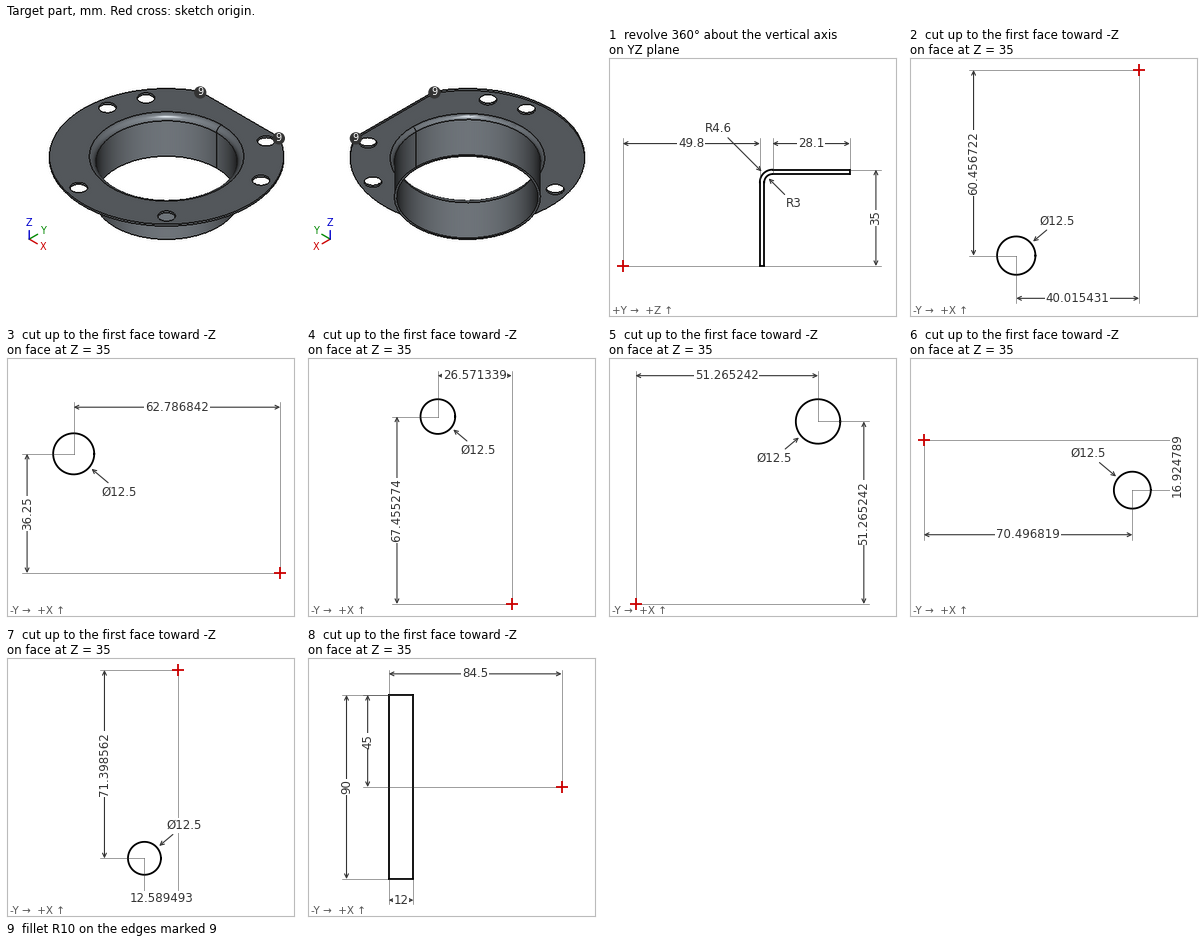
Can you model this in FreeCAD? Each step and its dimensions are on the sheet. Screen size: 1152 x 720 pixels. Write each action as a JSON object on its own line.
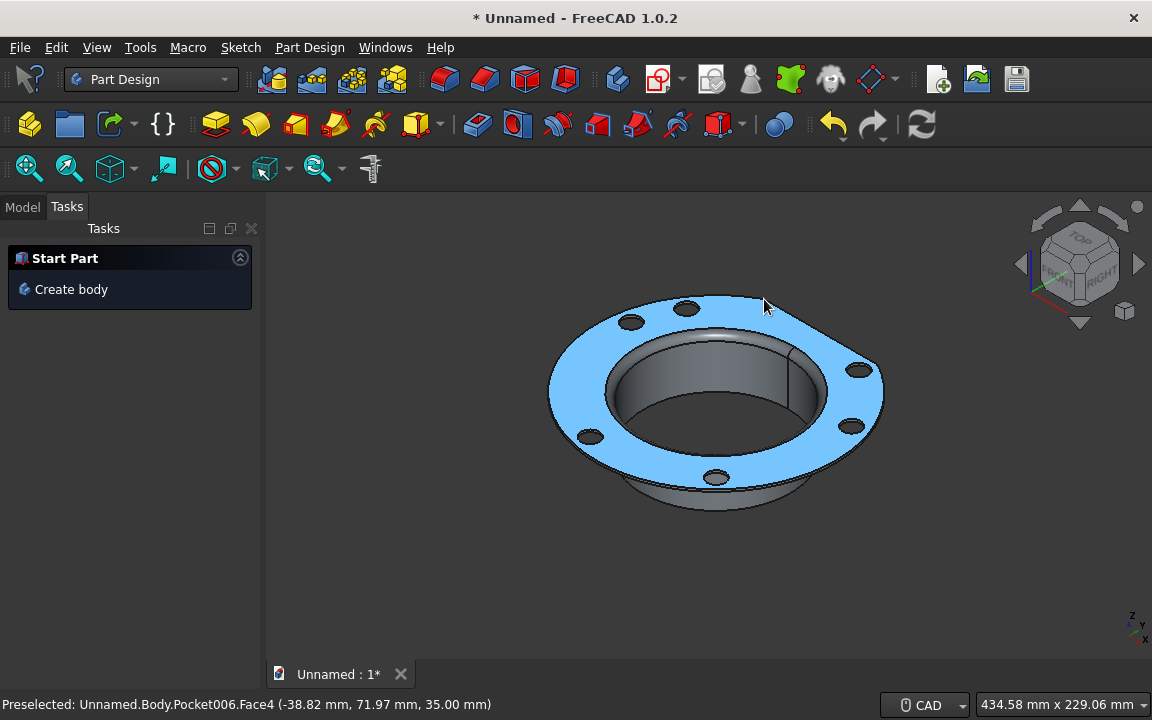
{"action": "key", "text": "2"}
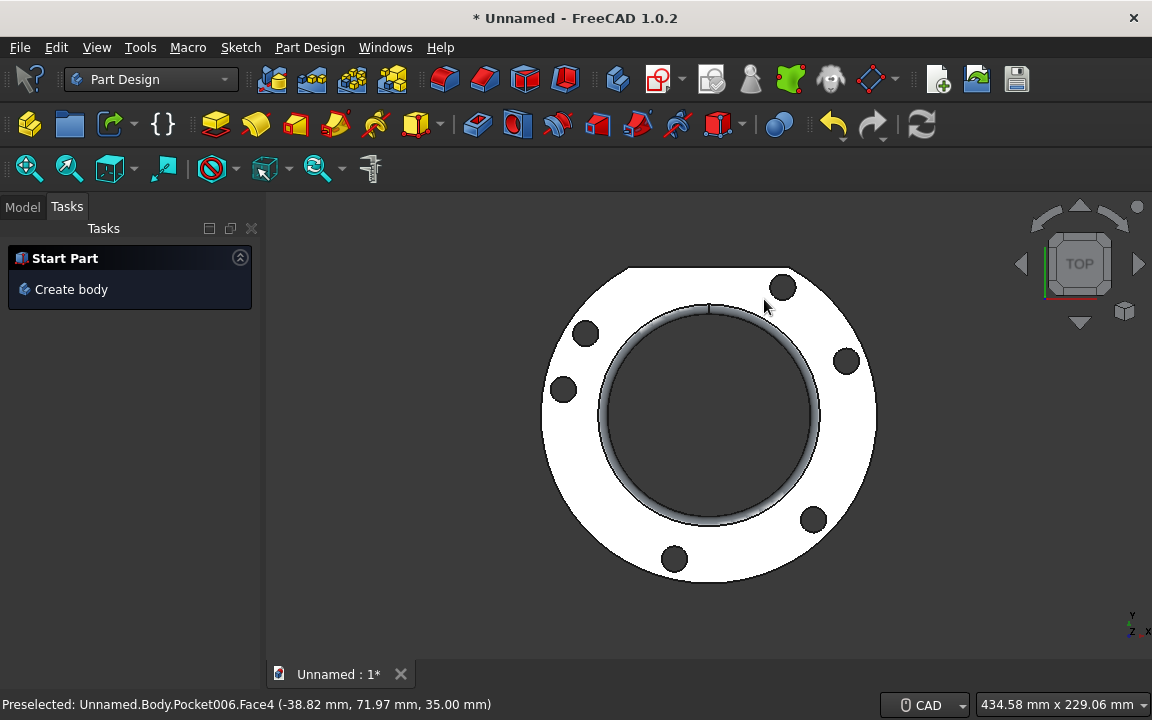
{"action": "scroll", "coordinate": [629, 266], "scroll_direction": "up", "scroll_amount": 13}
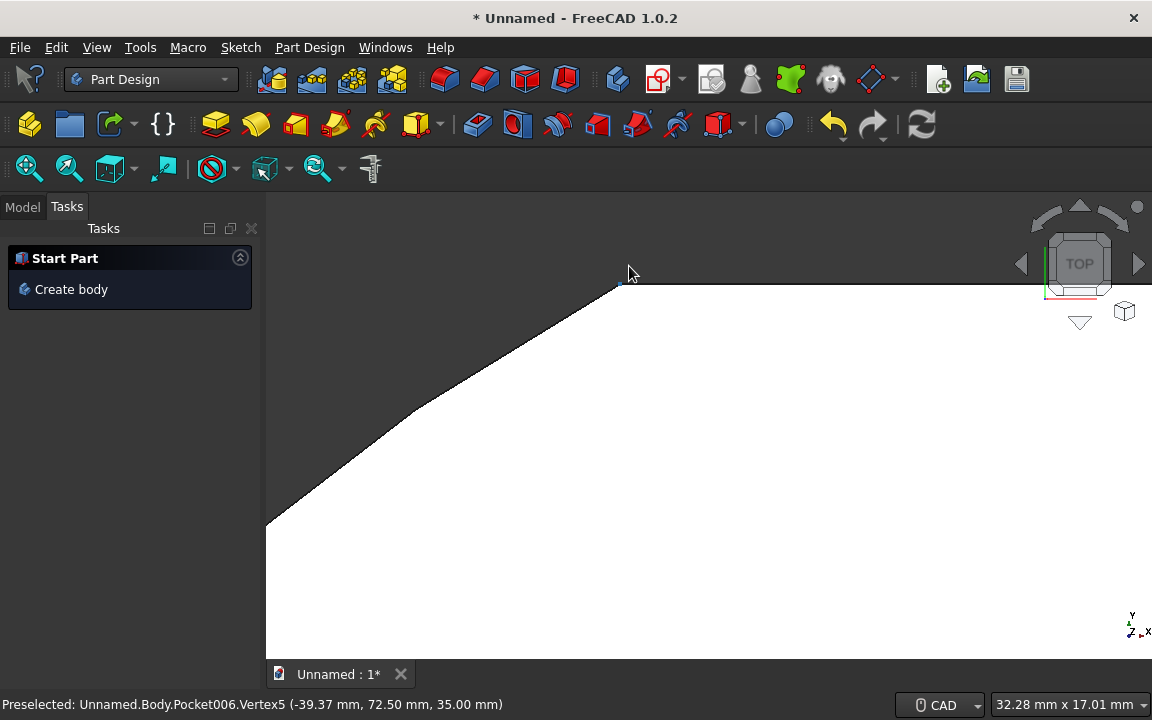
{"action": "key", "text": "v f"}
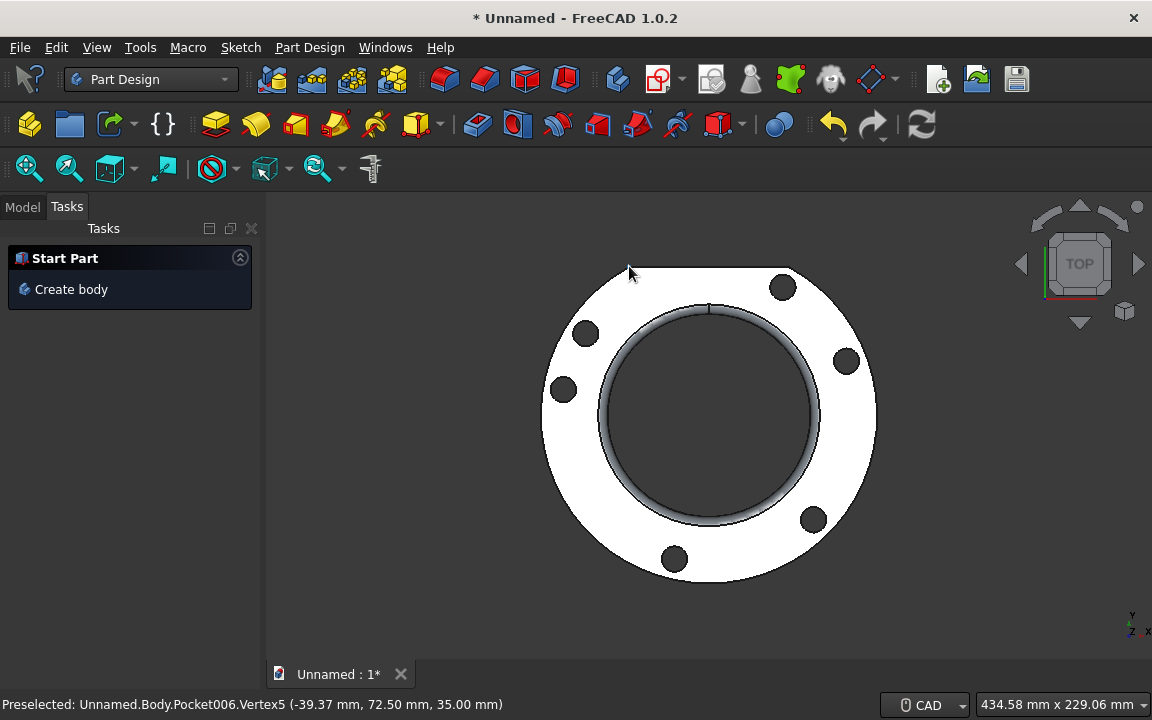
{"action": "key", "text": "1"}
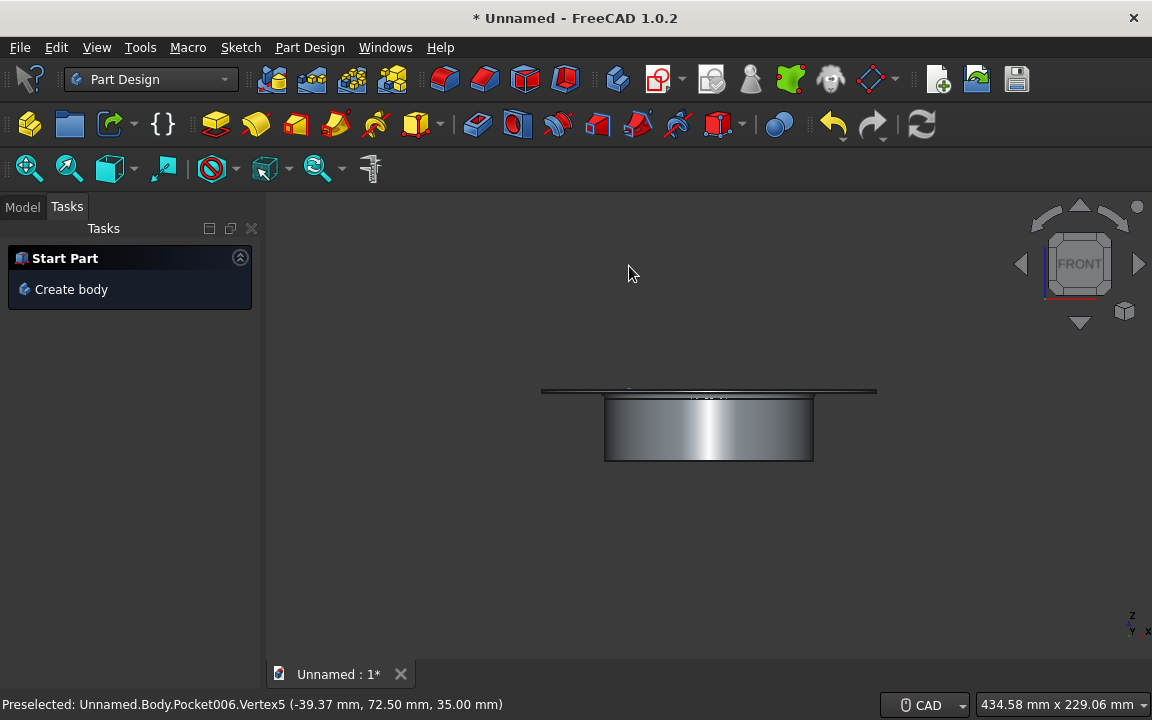
{"action": "left_click", "coordinate": [30, 170]}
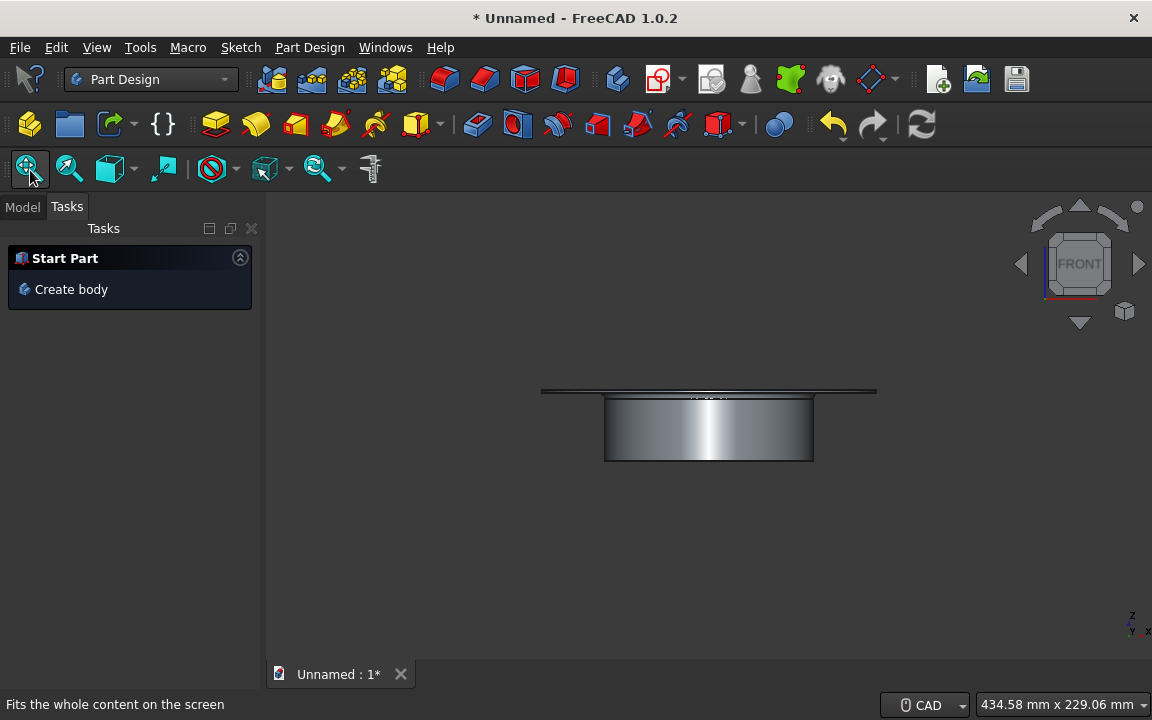
{"action": "scroll", "coordinate": [629, 390], "scroll_direction": "up", "scroll_amount": 13}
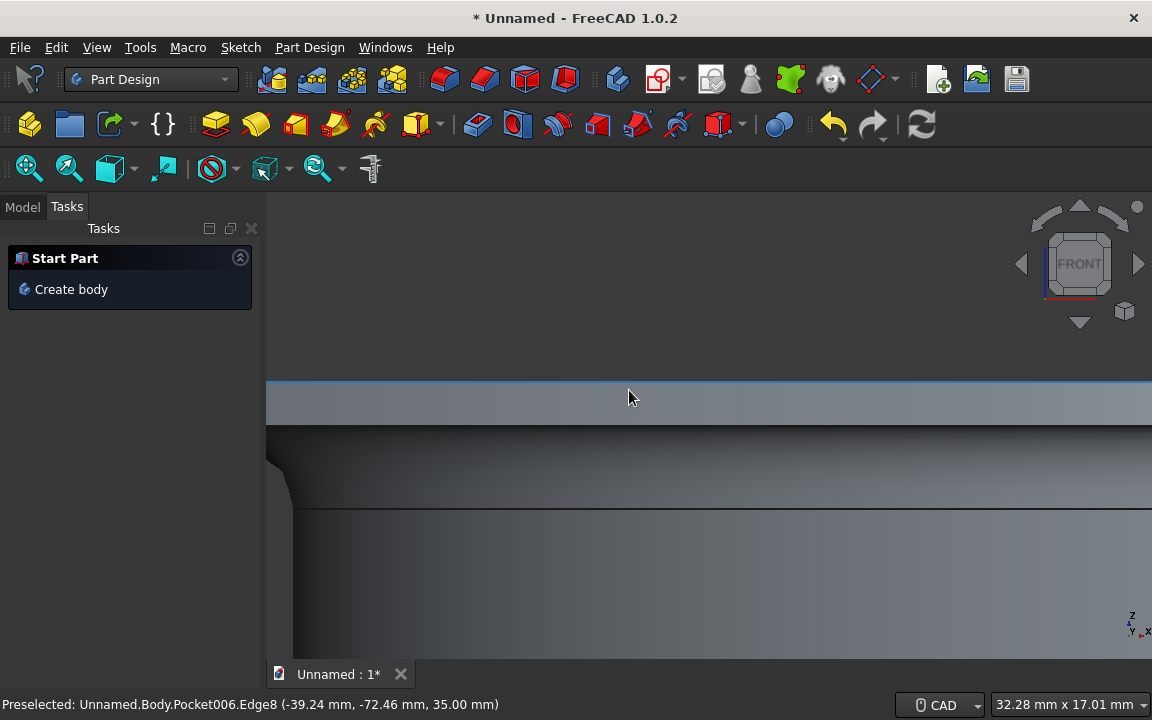
{"action": "key", "text": "v f"}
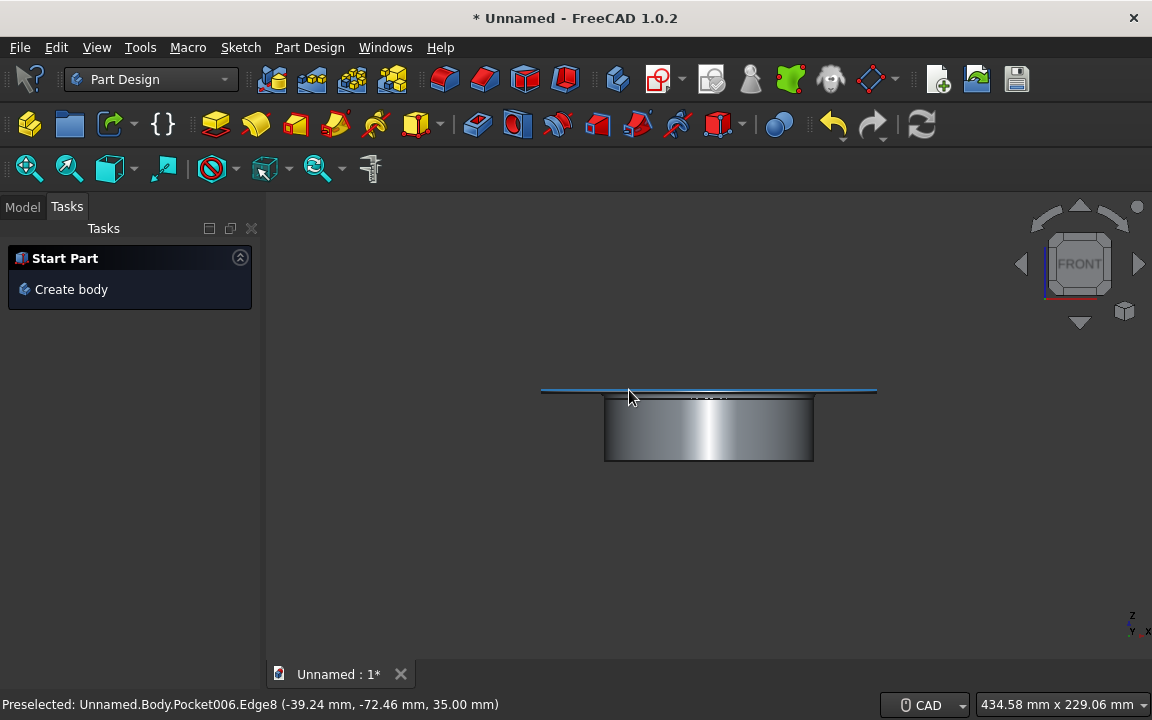
{"action": "key", "text": "3"}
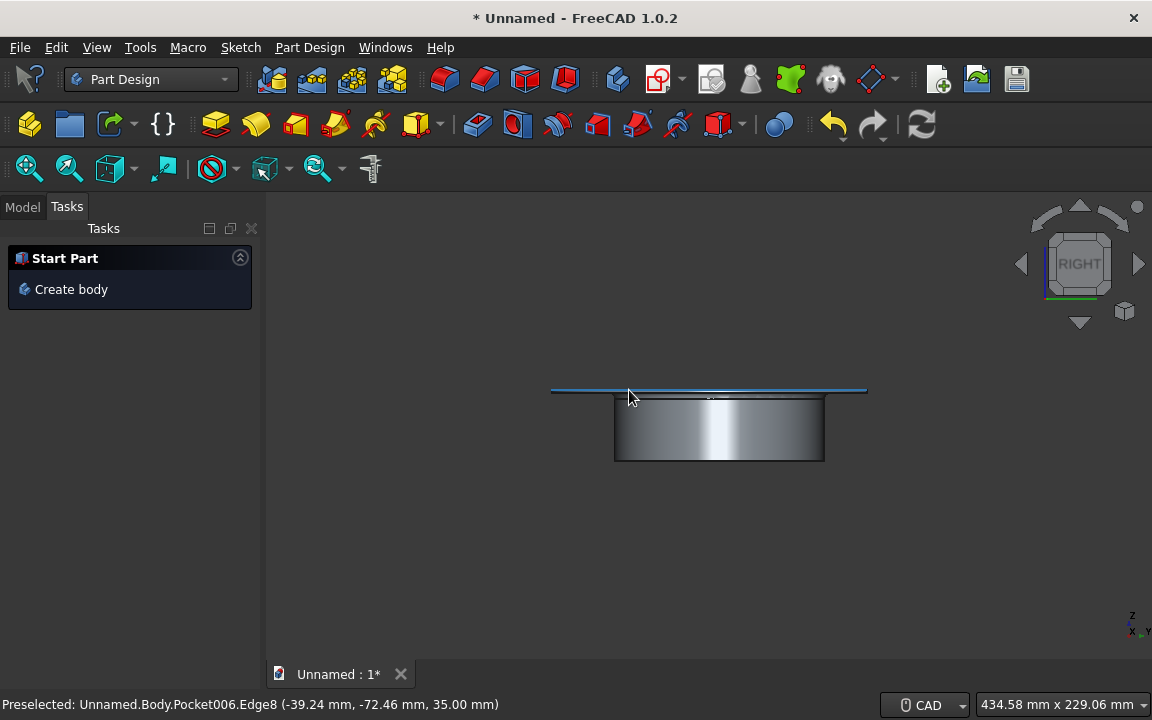
{"action": "key", "text": "v f"}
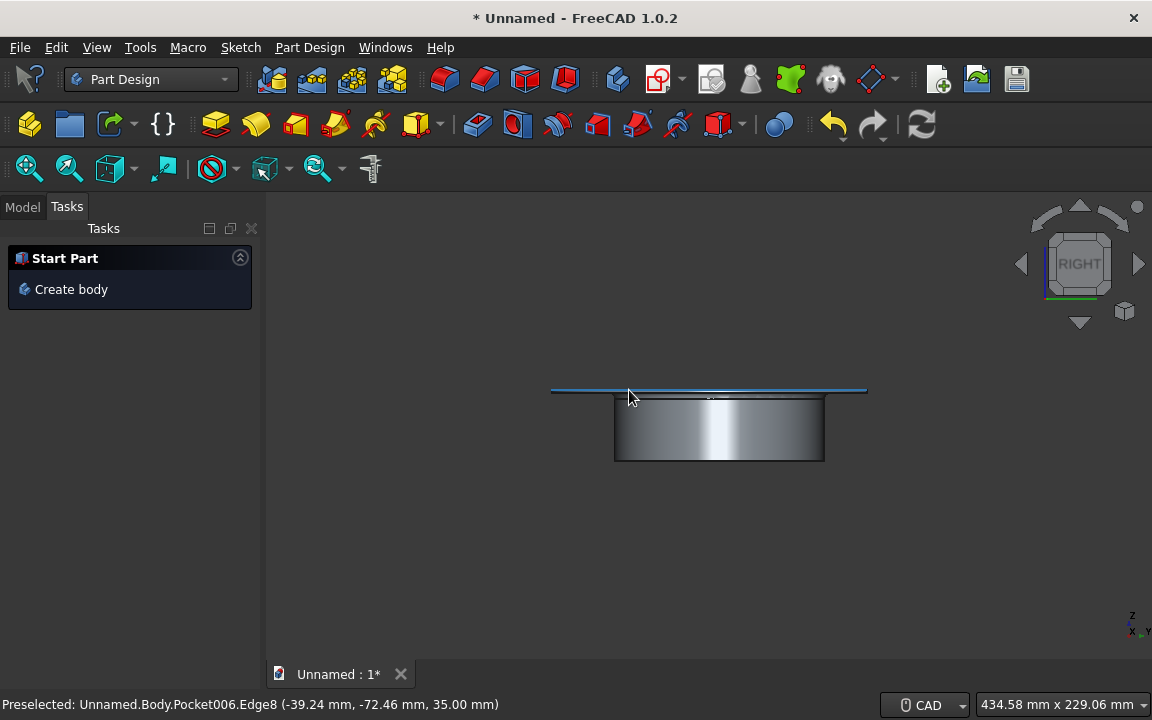
{"action": "scroll", "coordinate": [867, 390], "scroll_direction": "up", "scroll_amount": 13}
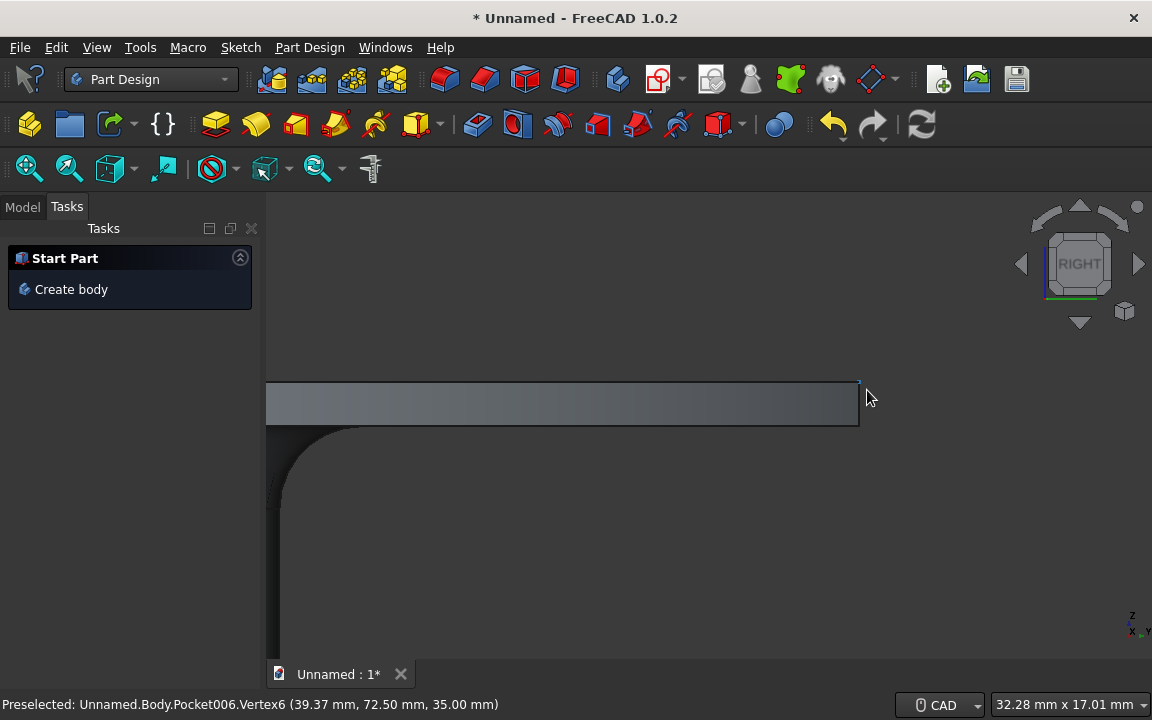
{"action": "key", "text": "v f"}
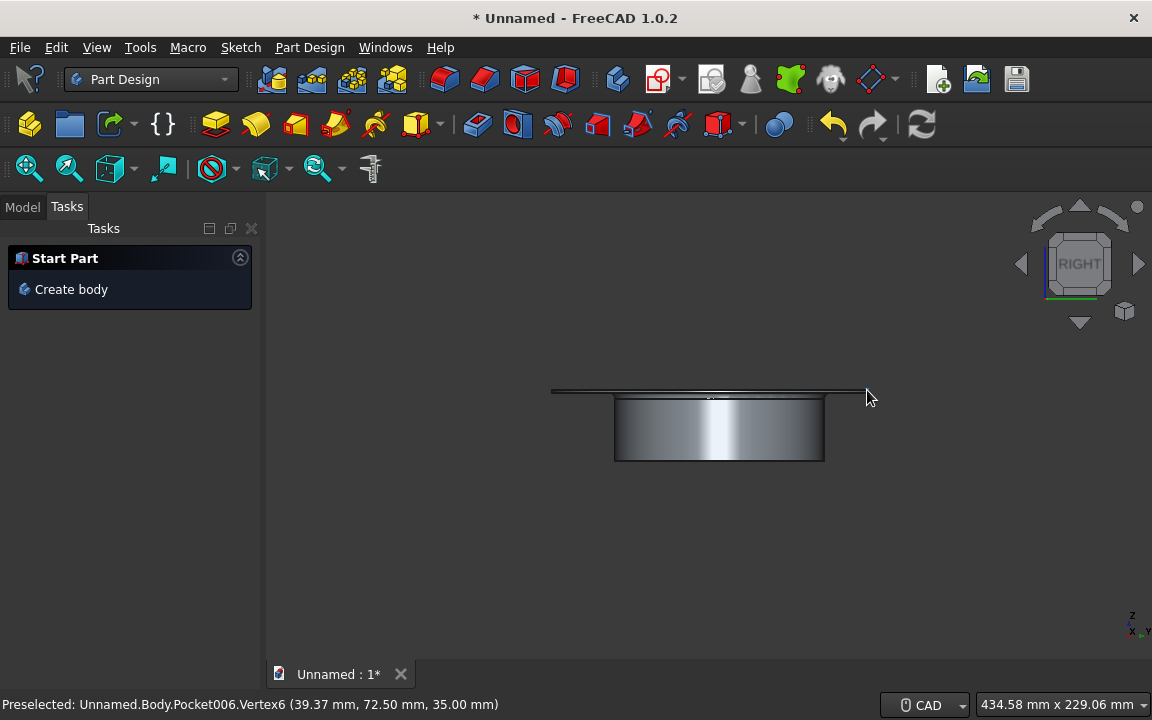
{"action": "key", "text": "5"}